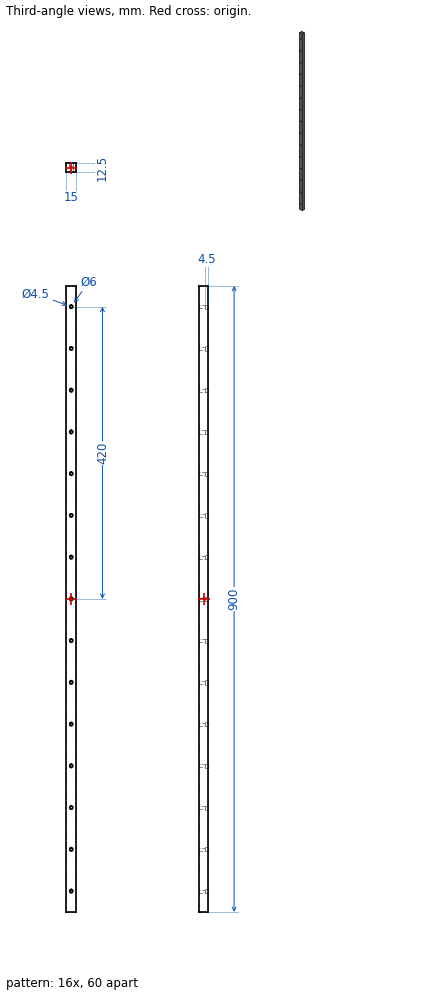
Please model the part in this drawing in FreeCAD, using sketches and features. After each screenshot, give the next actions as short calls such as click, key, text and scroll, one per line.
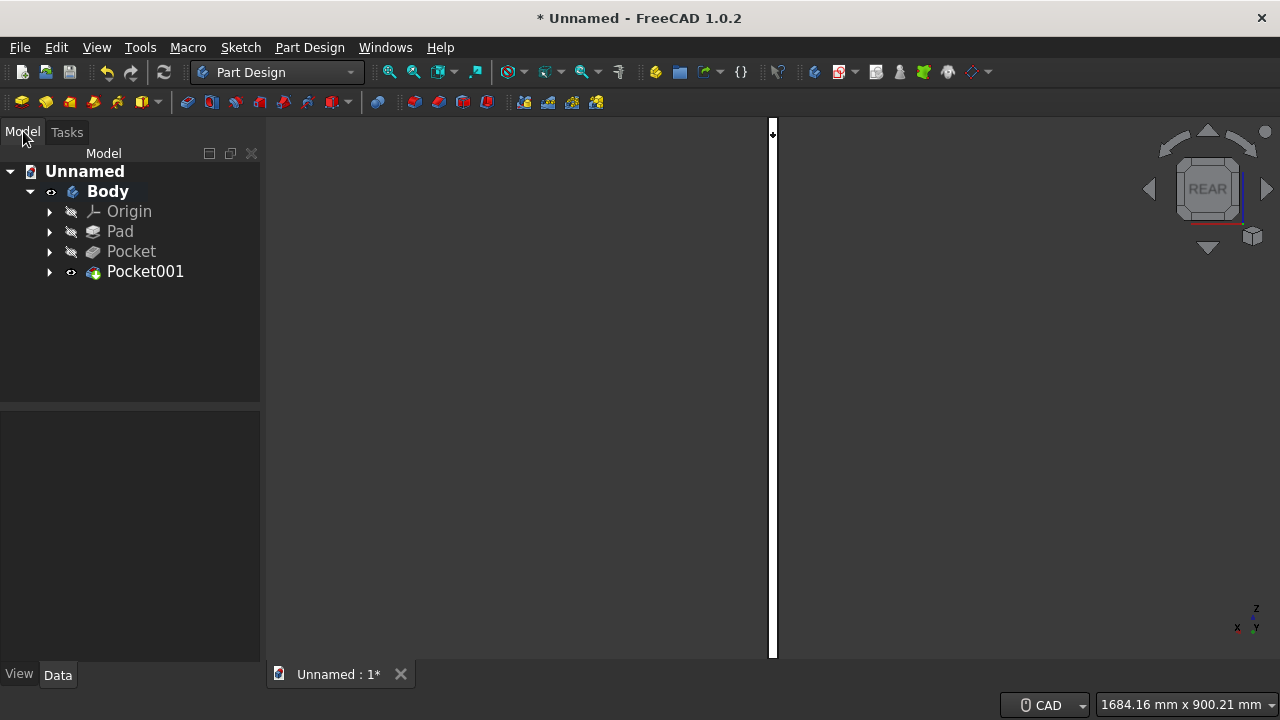
click(116, 252)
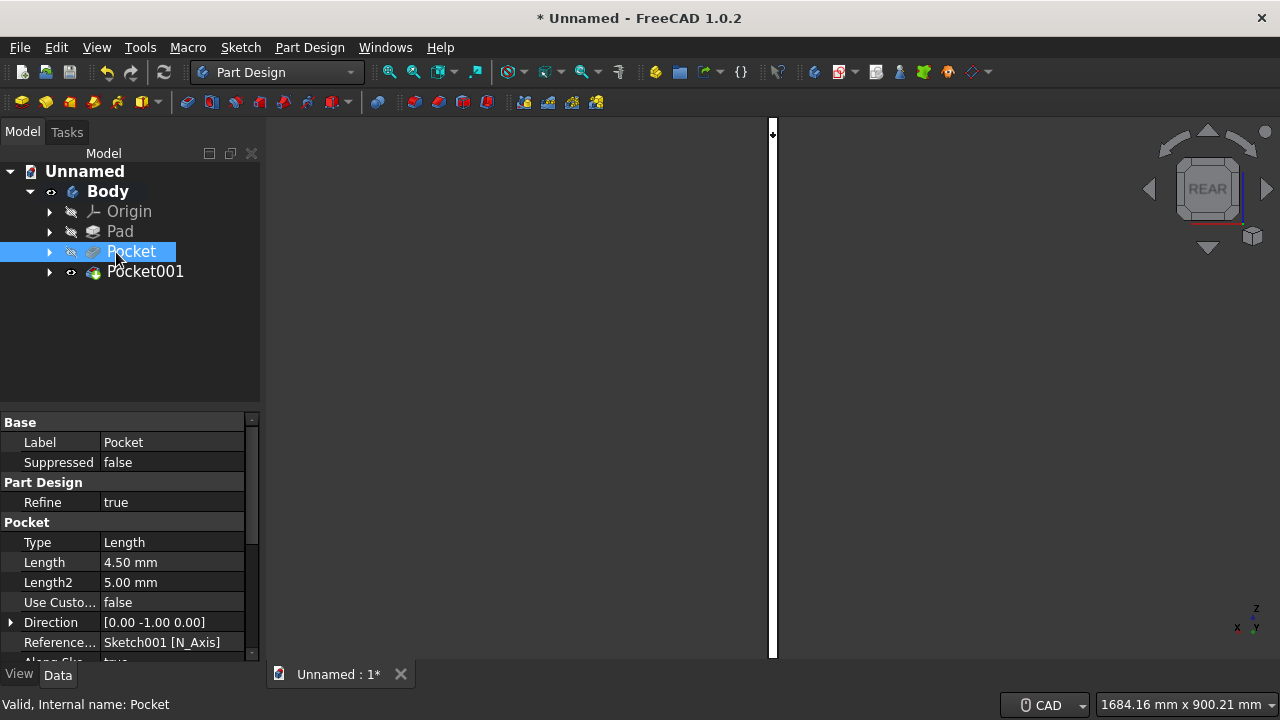
click(116, 272, ctrl)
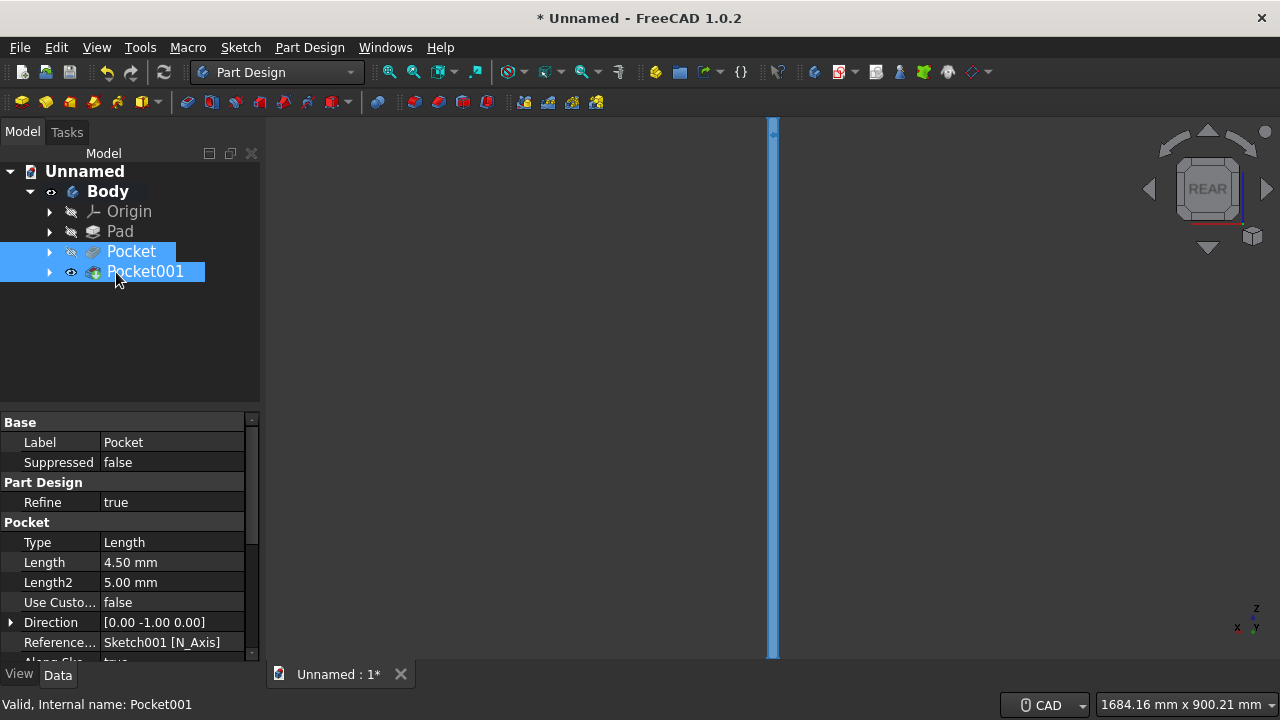
click(548, 102)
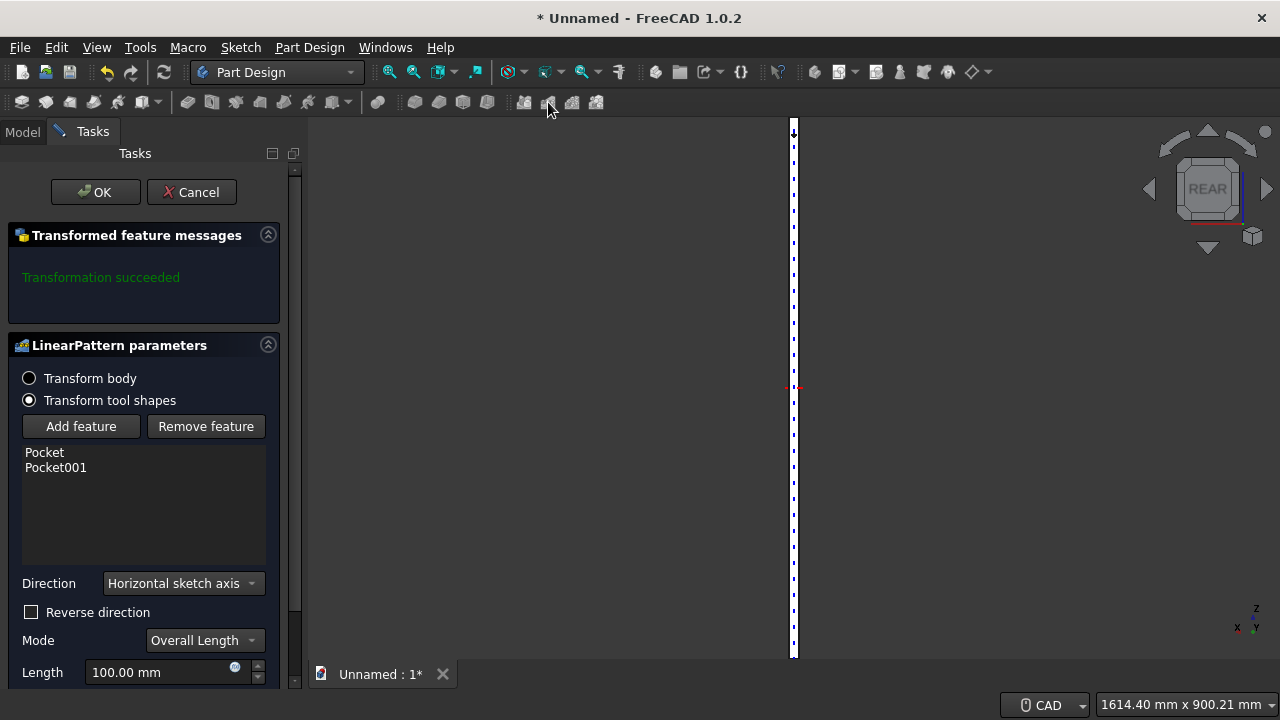
click(184, 584)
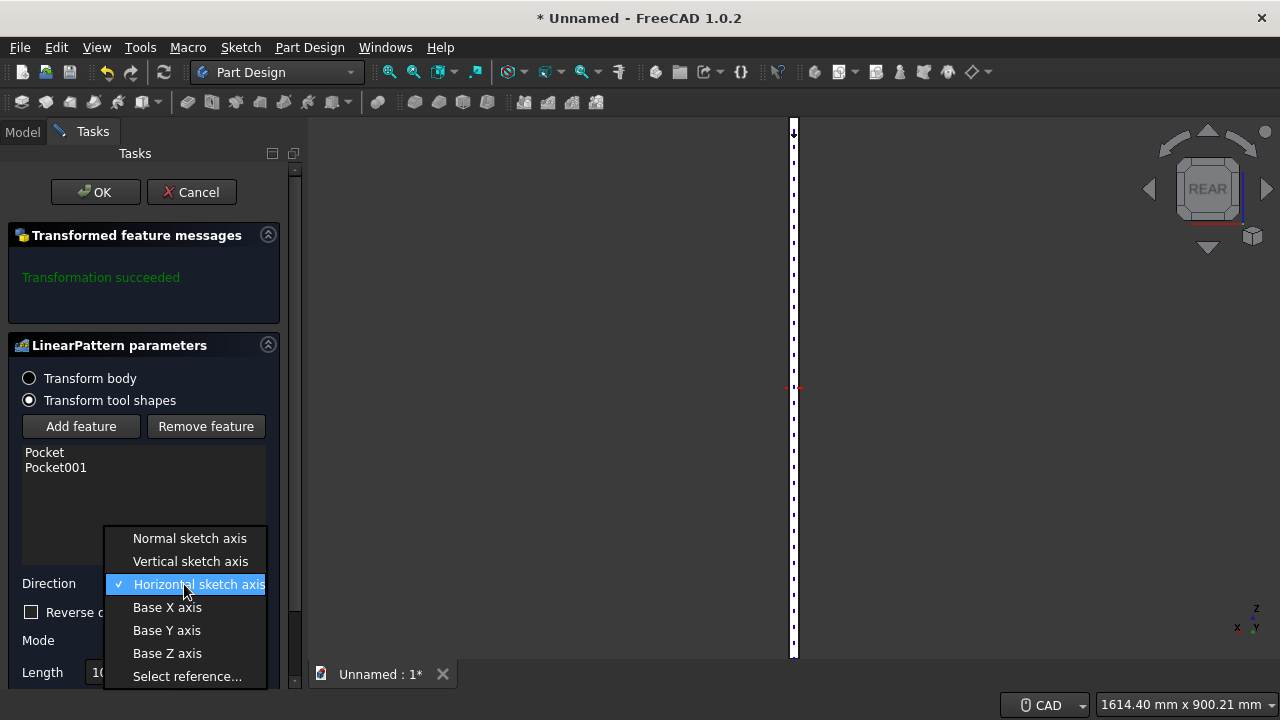
click(184, 654)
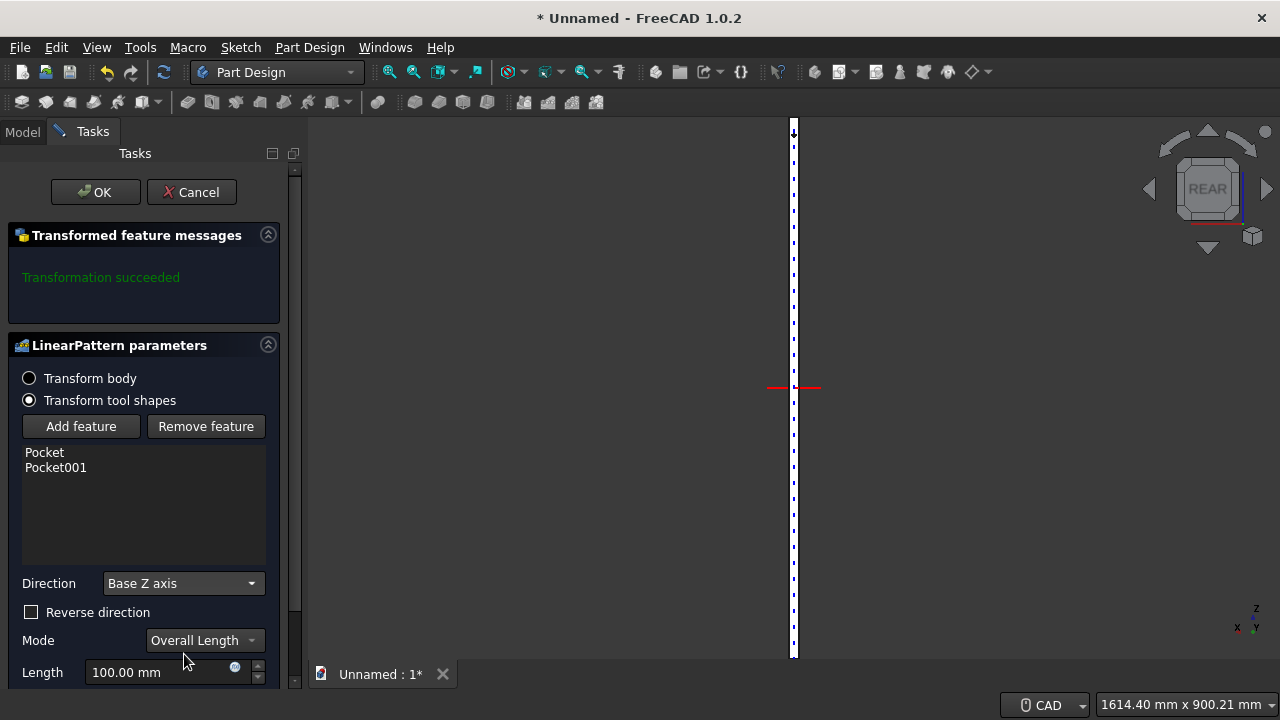
click(206, 640)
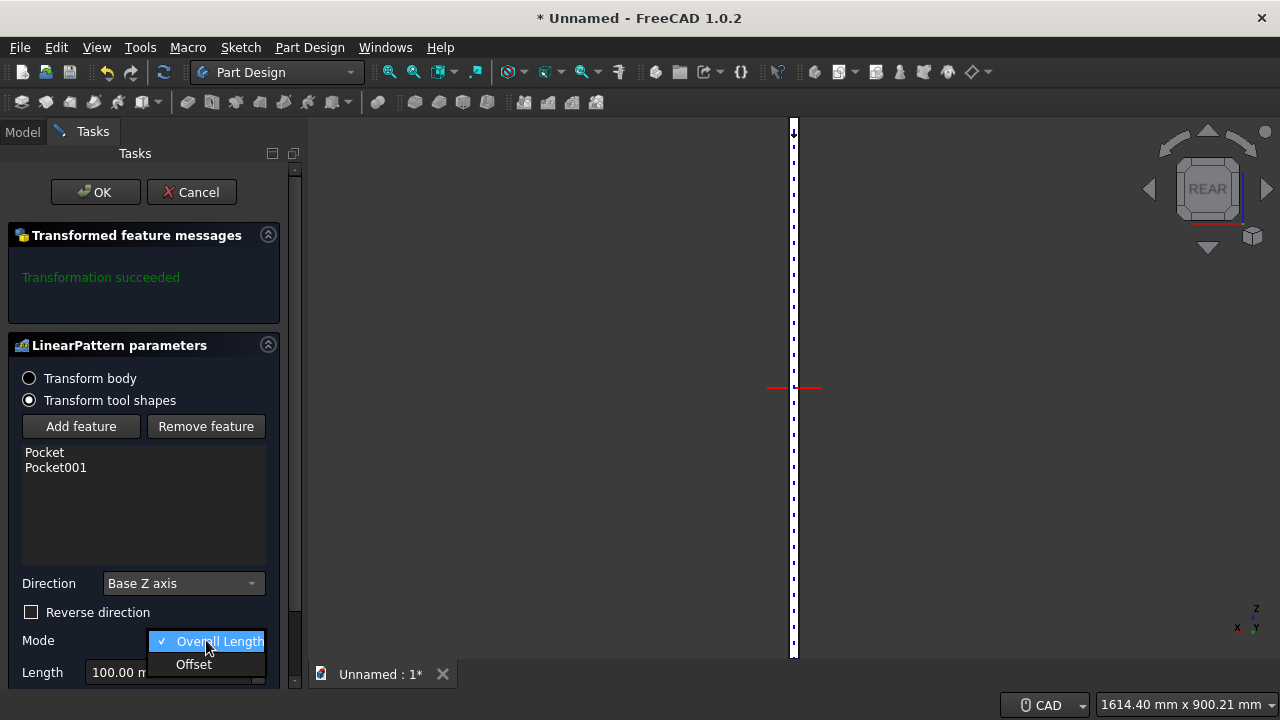
click(206, 664)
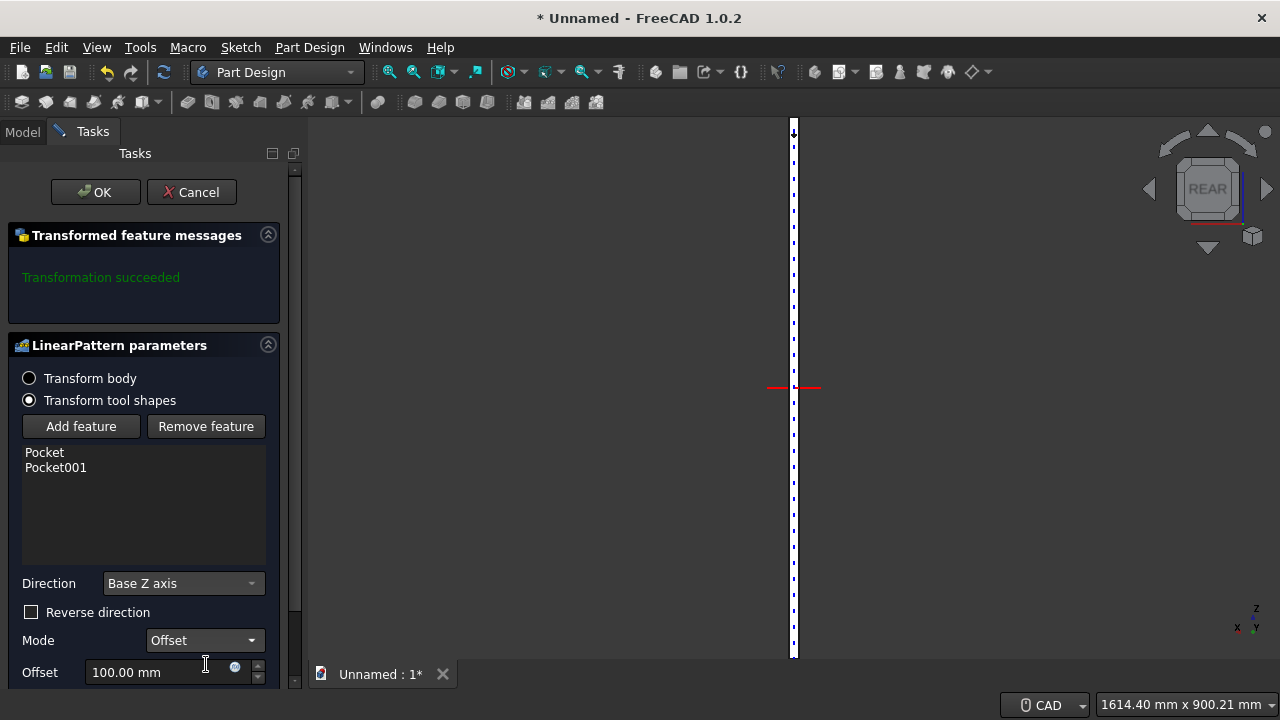
triple_click(168, 672)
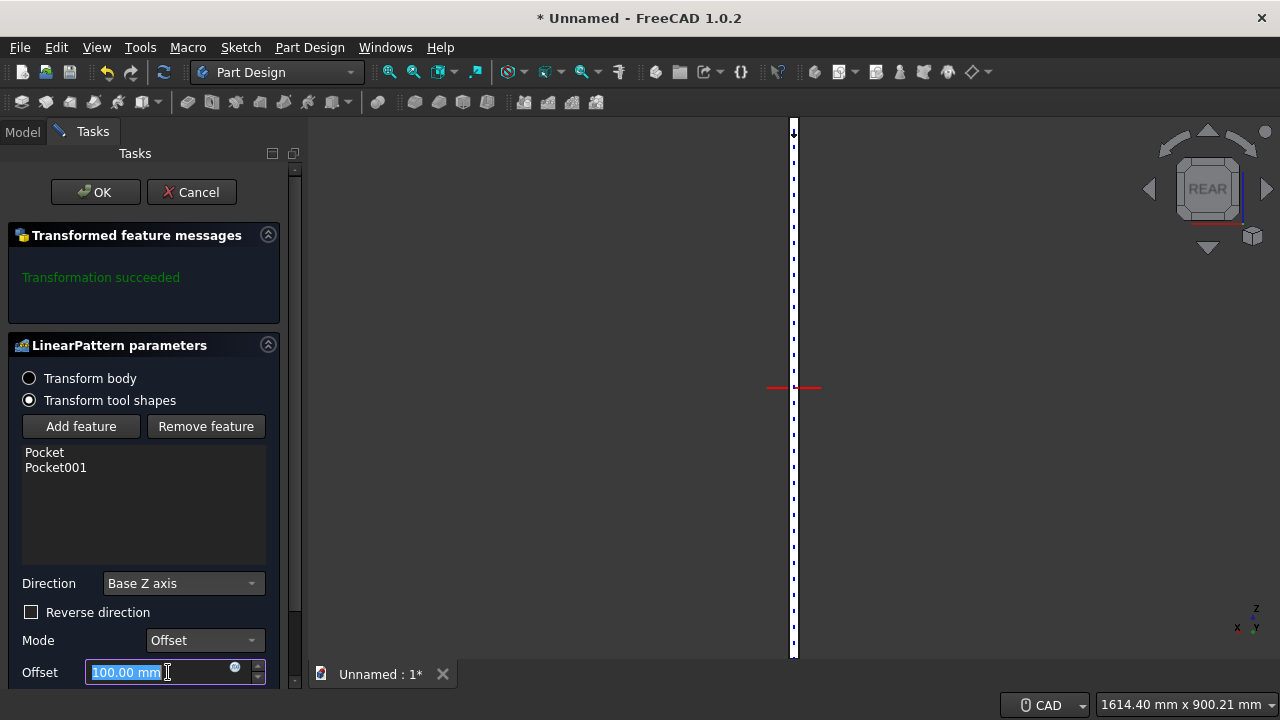
text(60)
key(Tab)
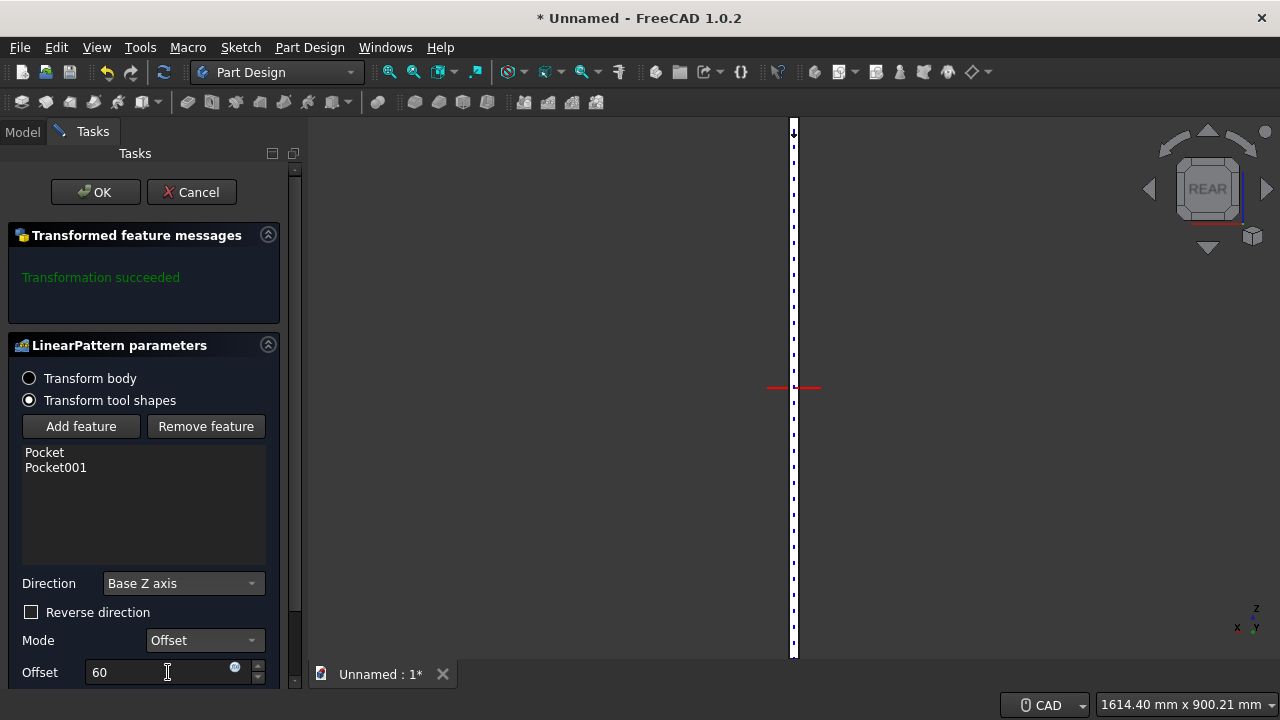
scroll(295, 426, down, 2)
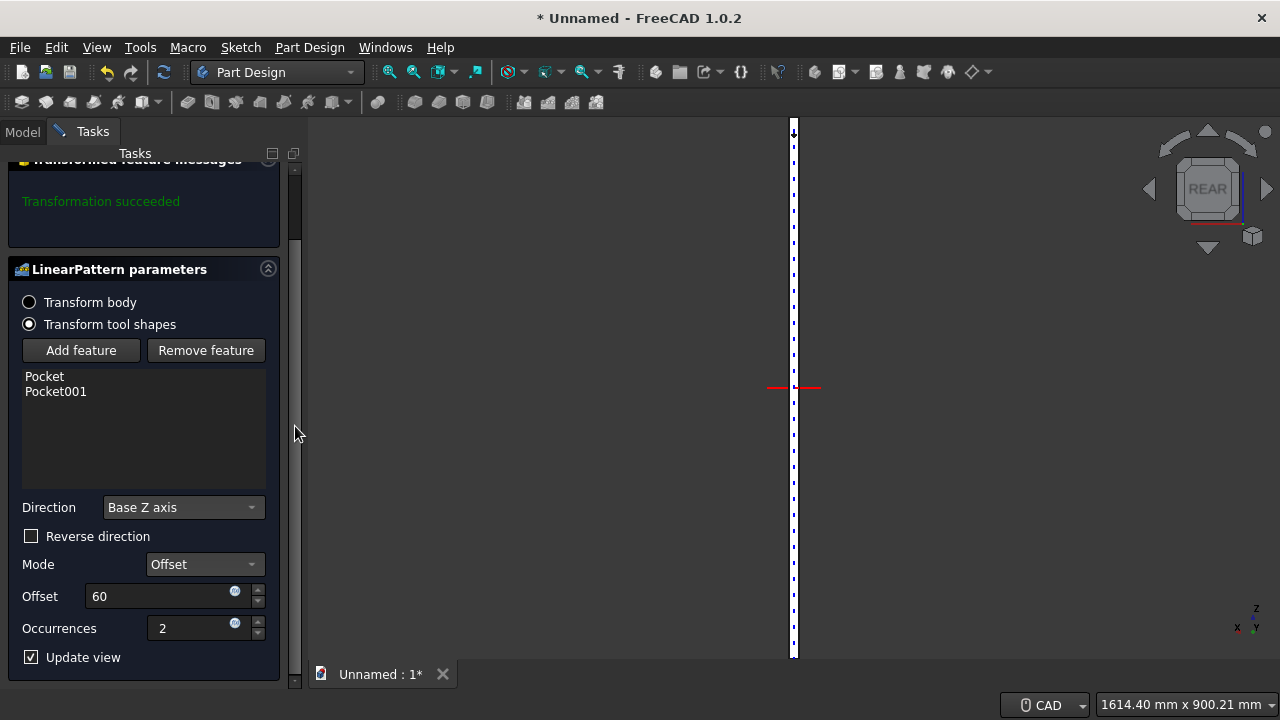
triple_click(198, 628)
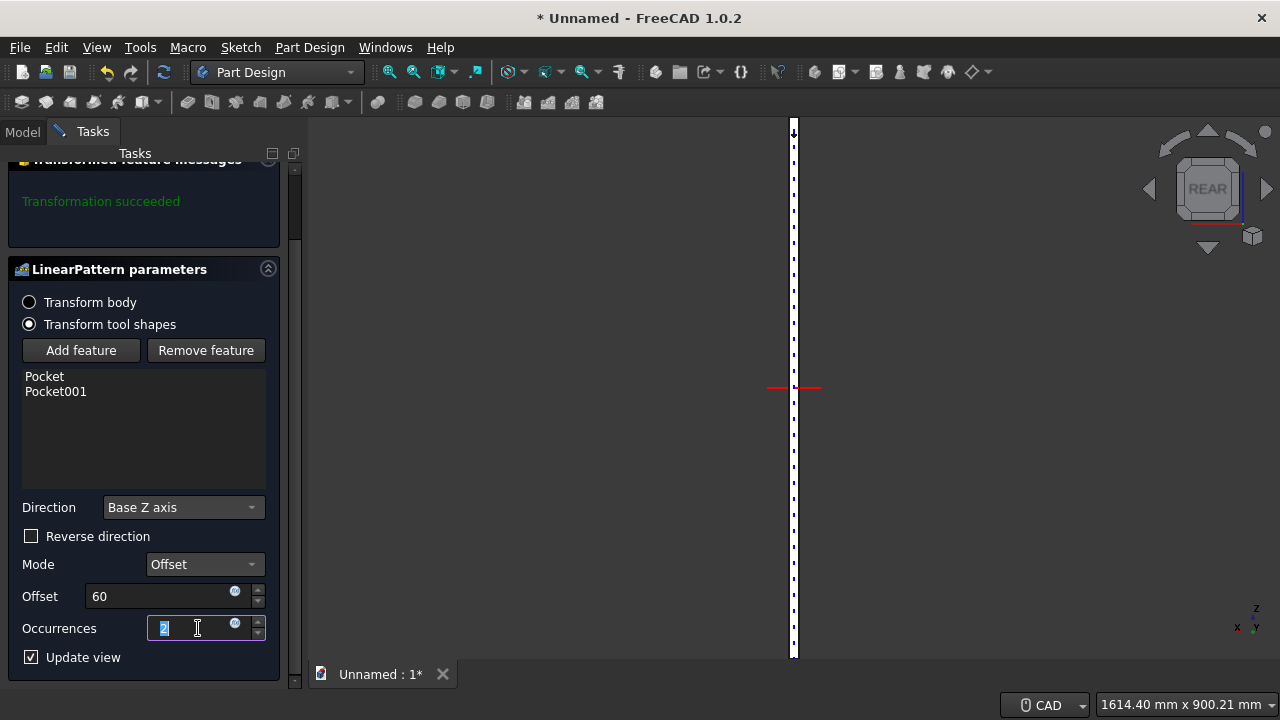
text(16)
key(Tab)